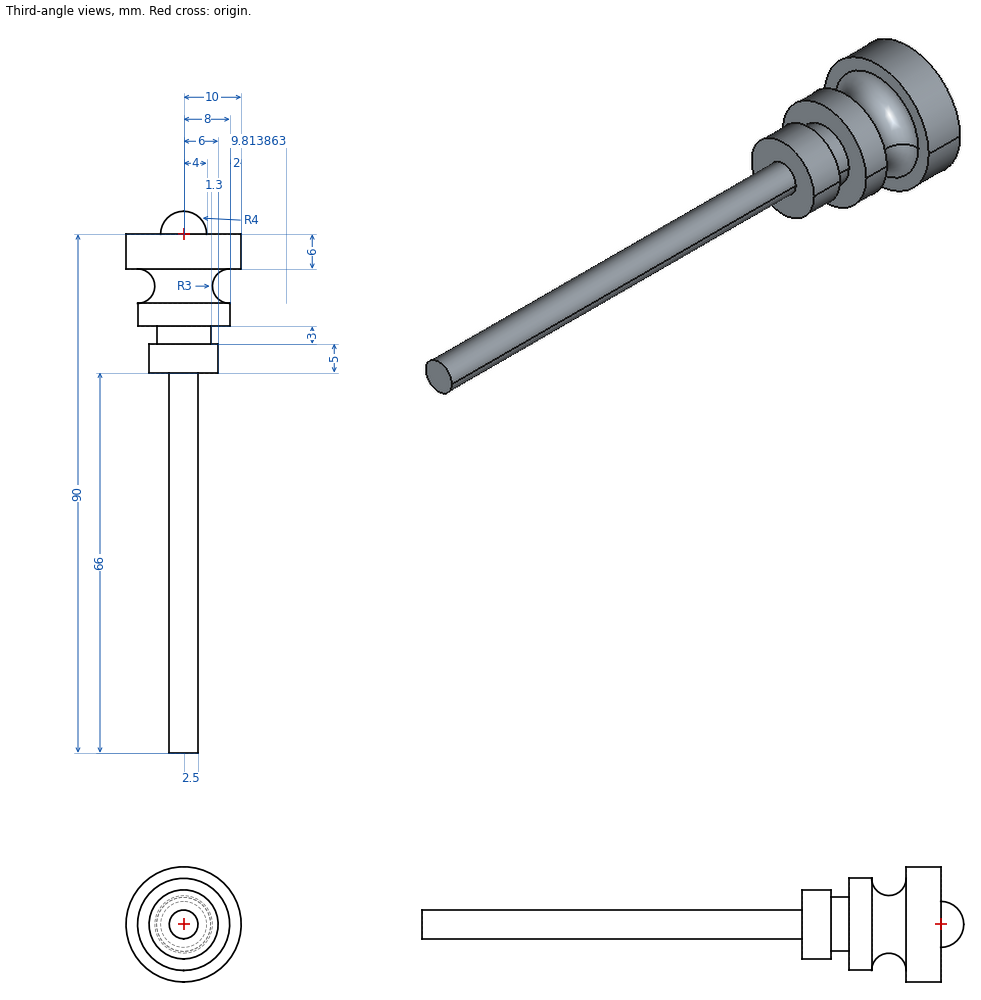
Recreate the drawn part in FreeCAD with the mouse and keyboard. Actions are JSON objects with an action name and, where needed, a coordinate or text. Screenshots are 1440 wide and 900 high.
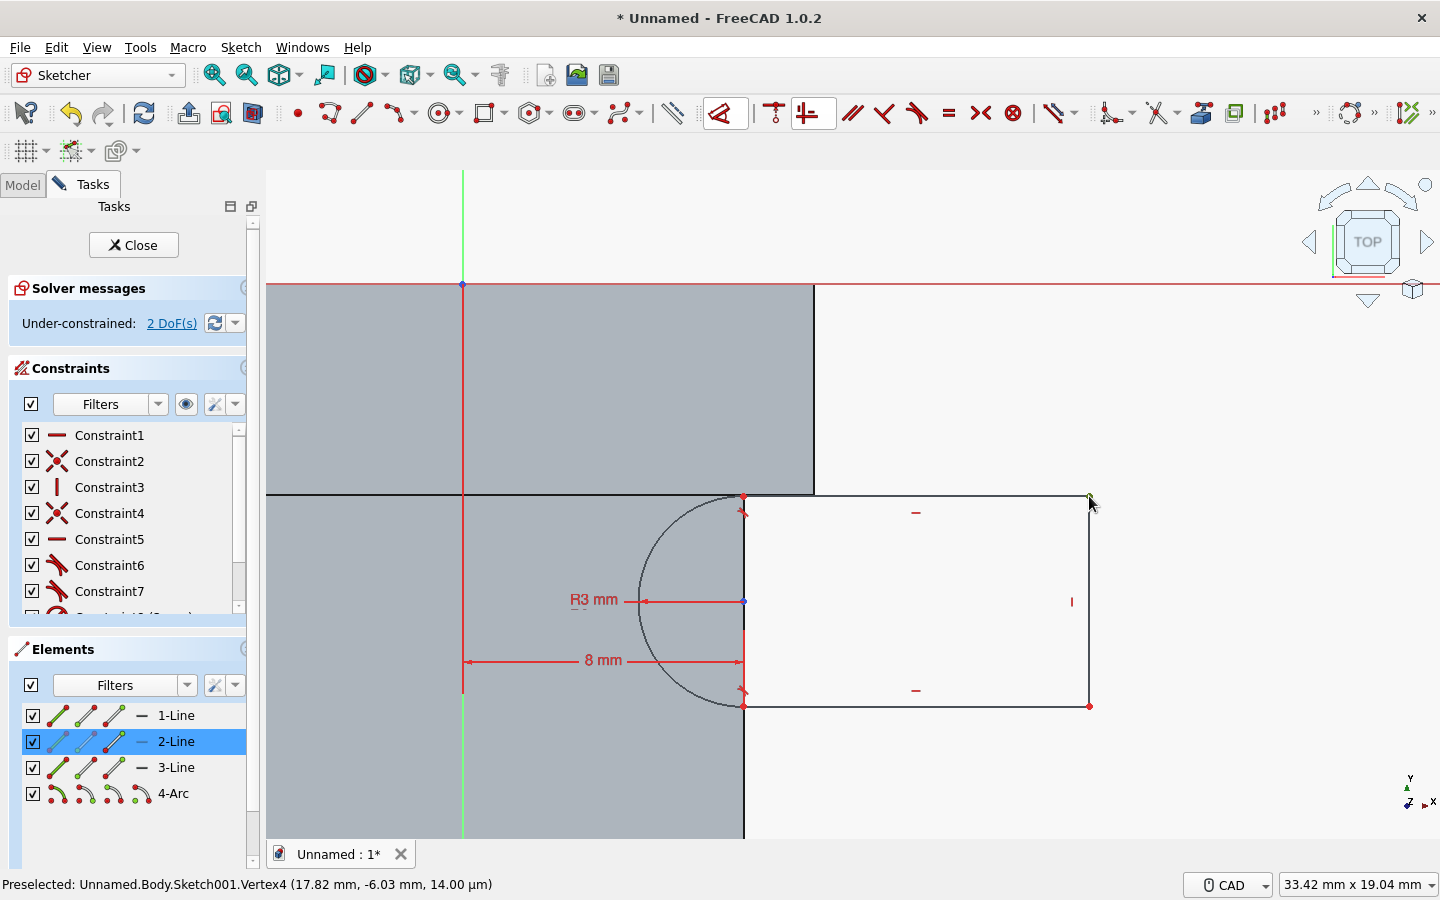
{"action": "key", "text": "i"}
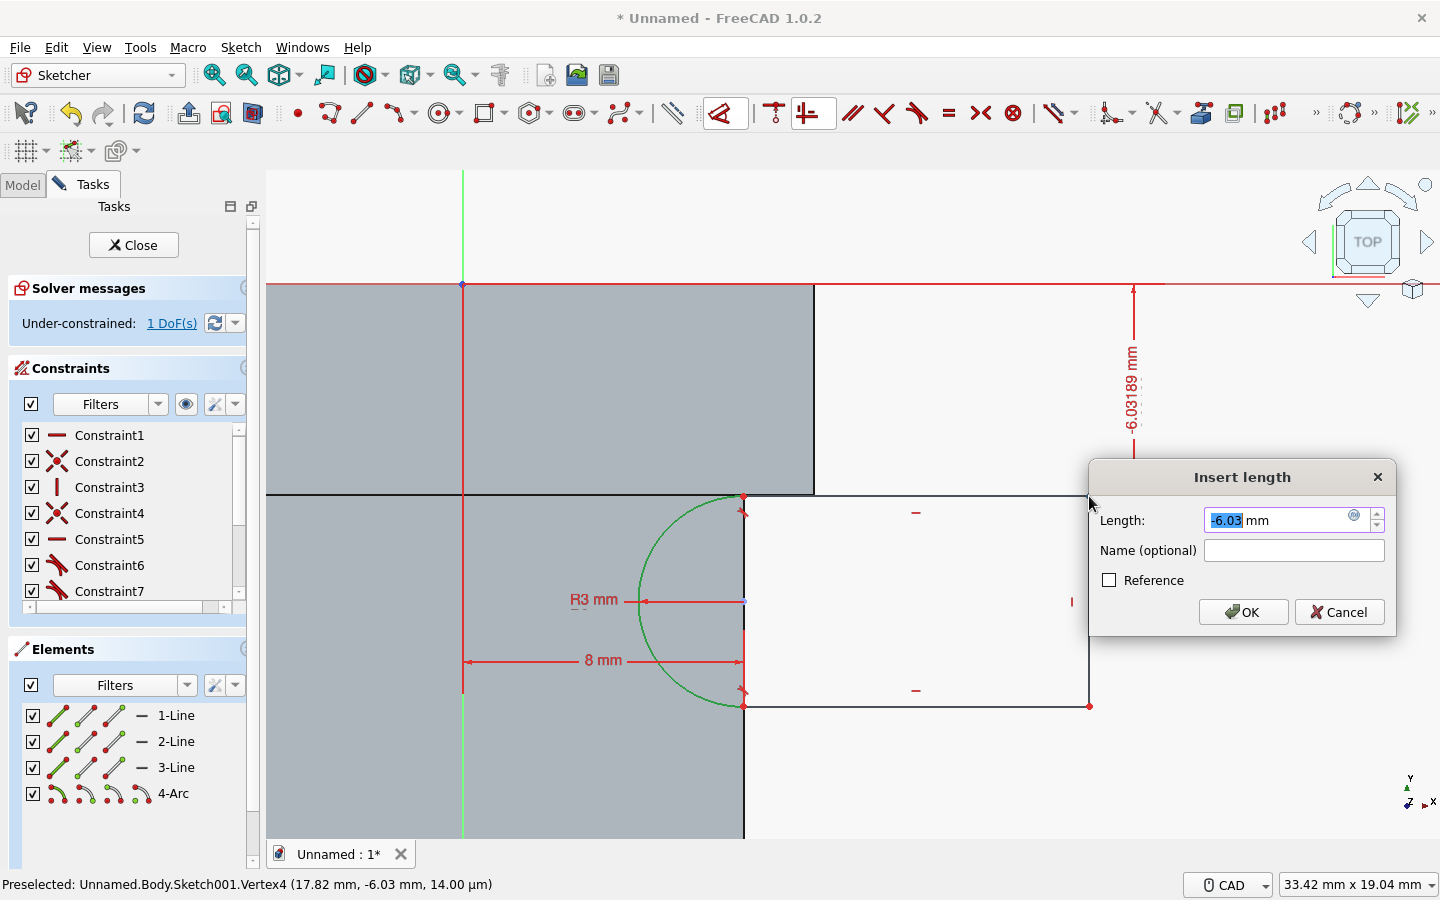
{"action": "type", "text": "-6"}
{"action": "key", "text": "Return"}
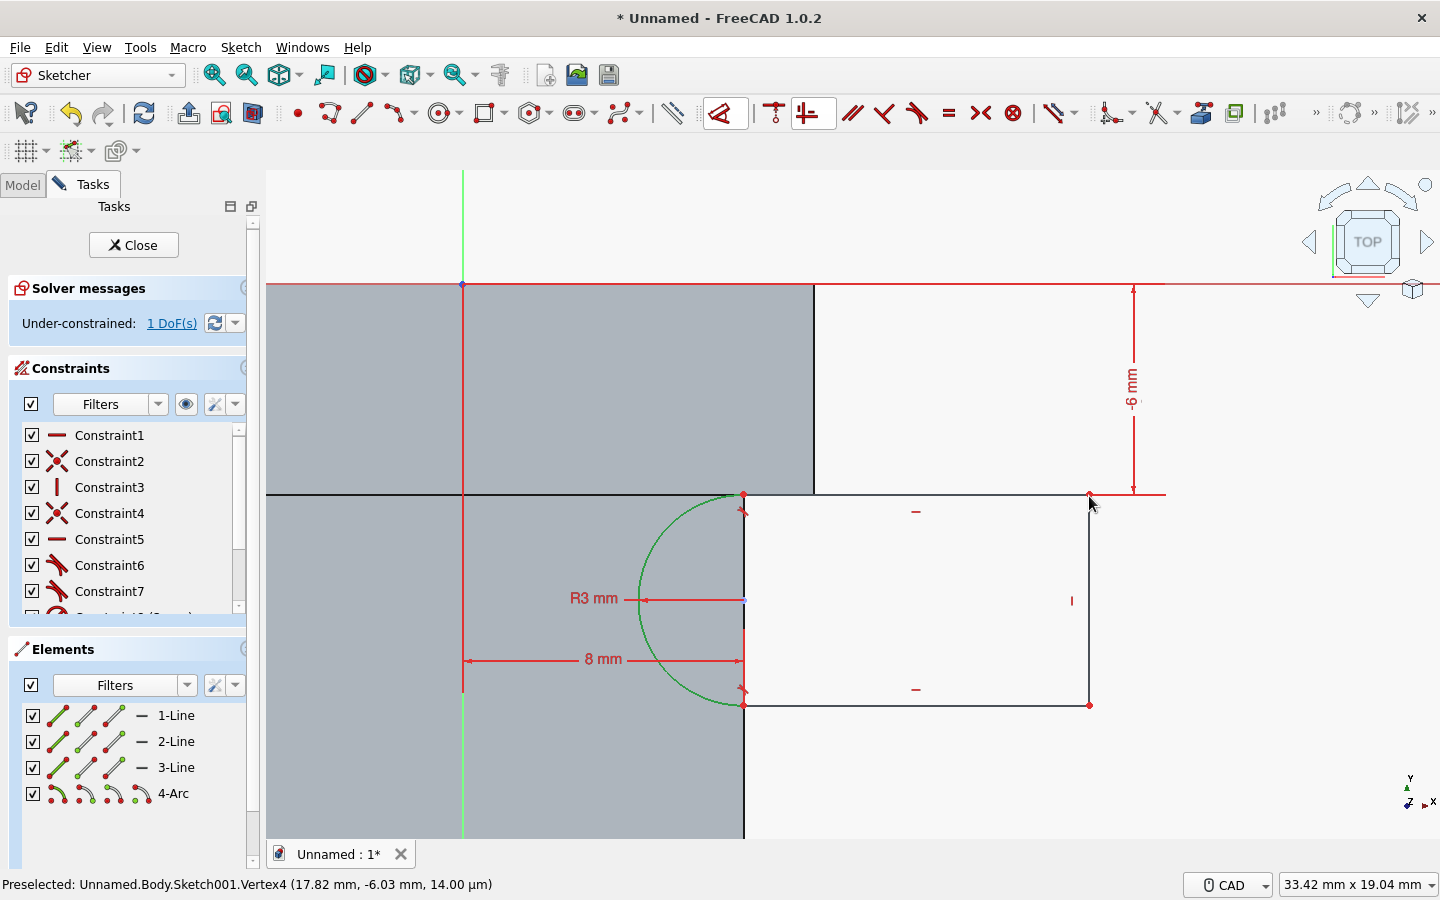
{"action": "left_click", "coordinate": [847, 706]}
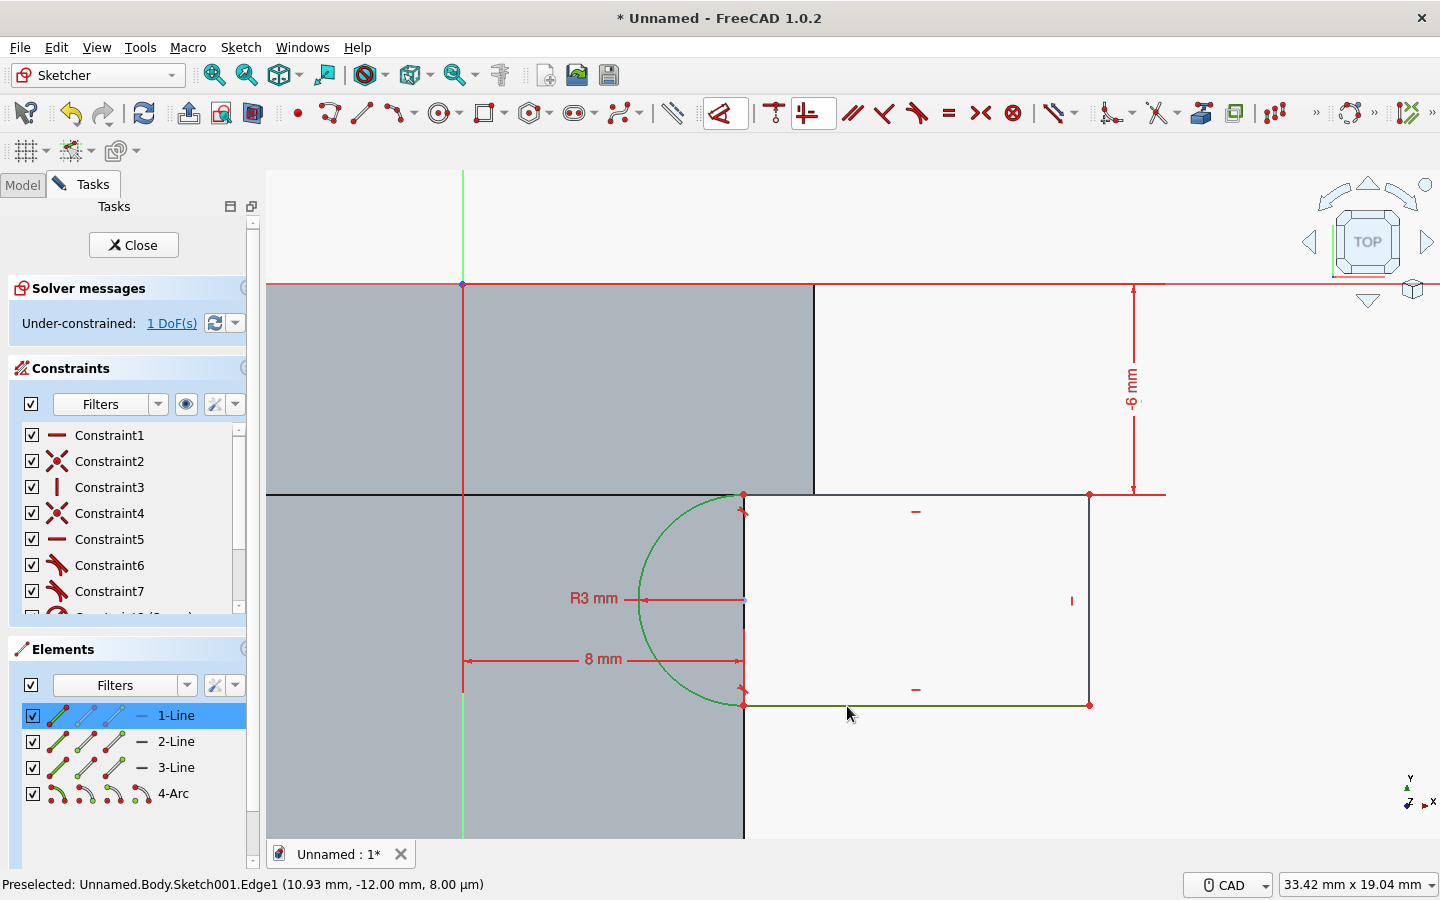
{"action": "key", "text": "l"}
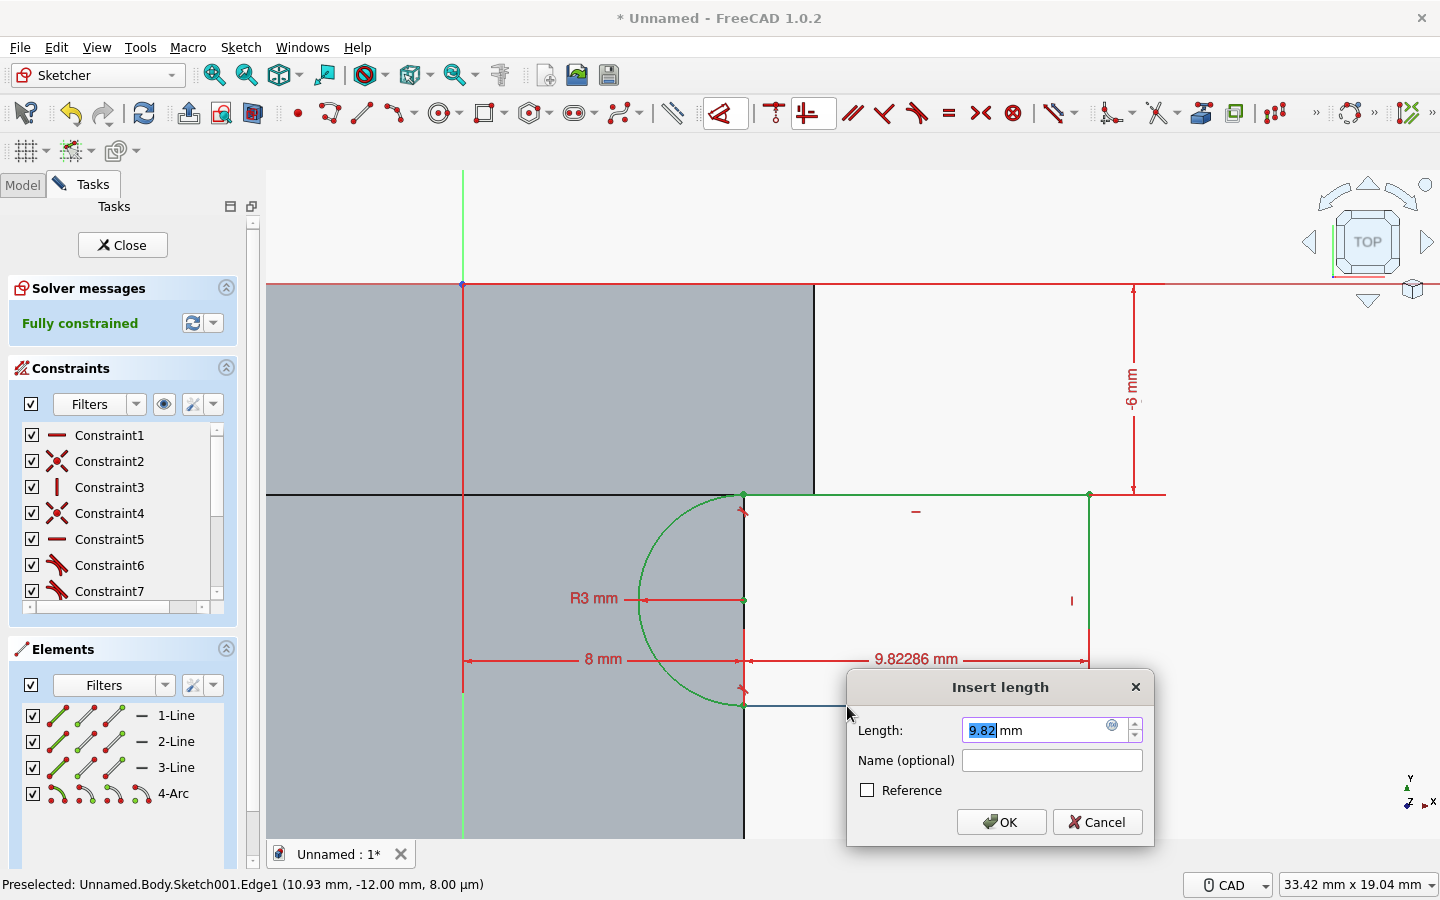
{"action": "type", "text": "9.813863"}
{"action": "key", "text": "Return"}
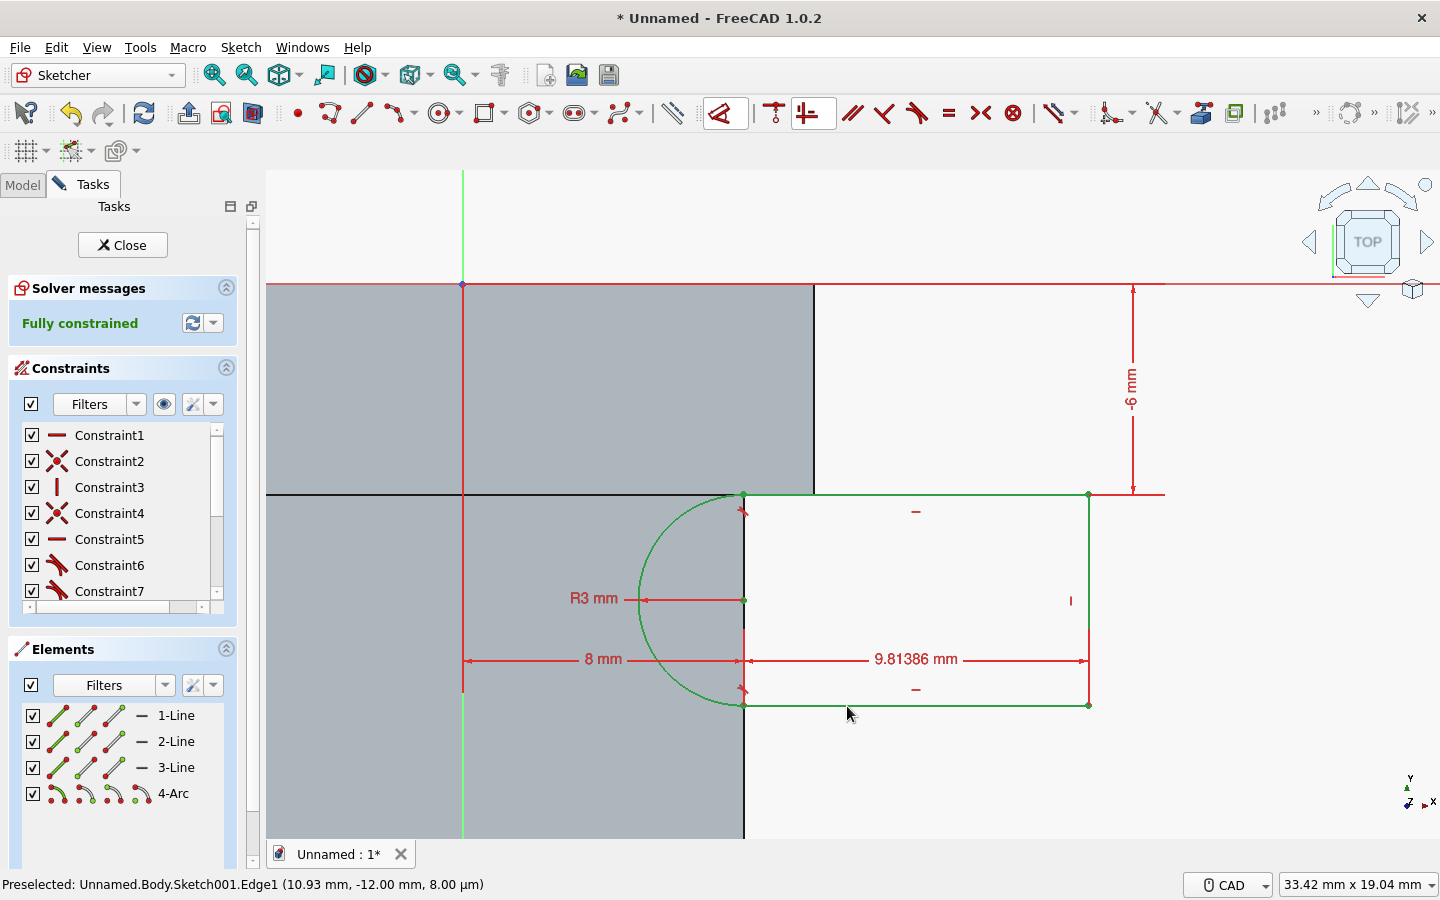
{"action": "left_click", "coordinate": [123, 245]}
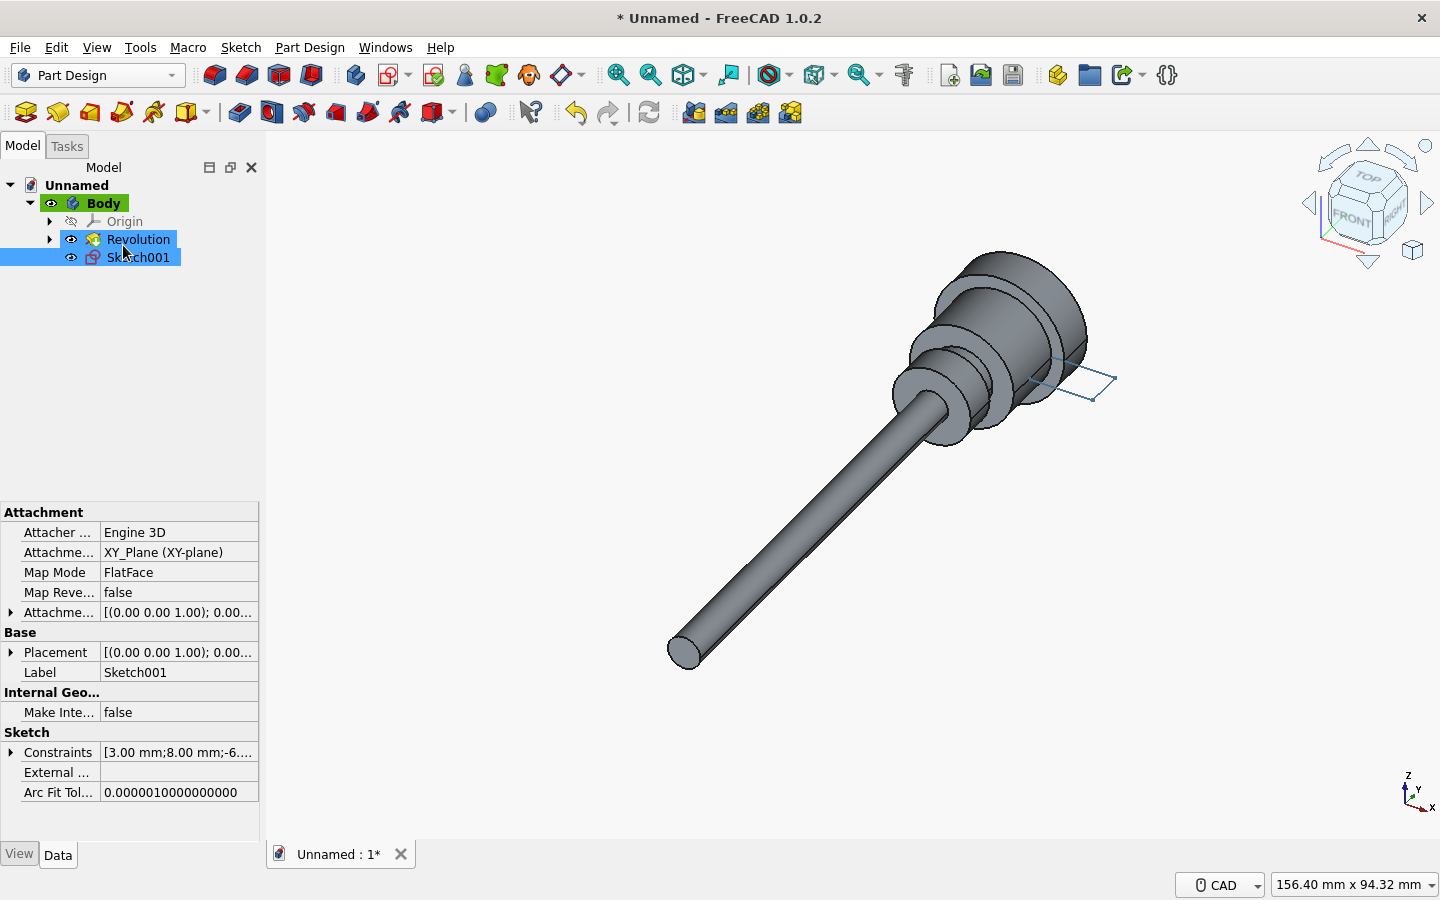
{"action": "left_click", "coordinate": [304, 112]}